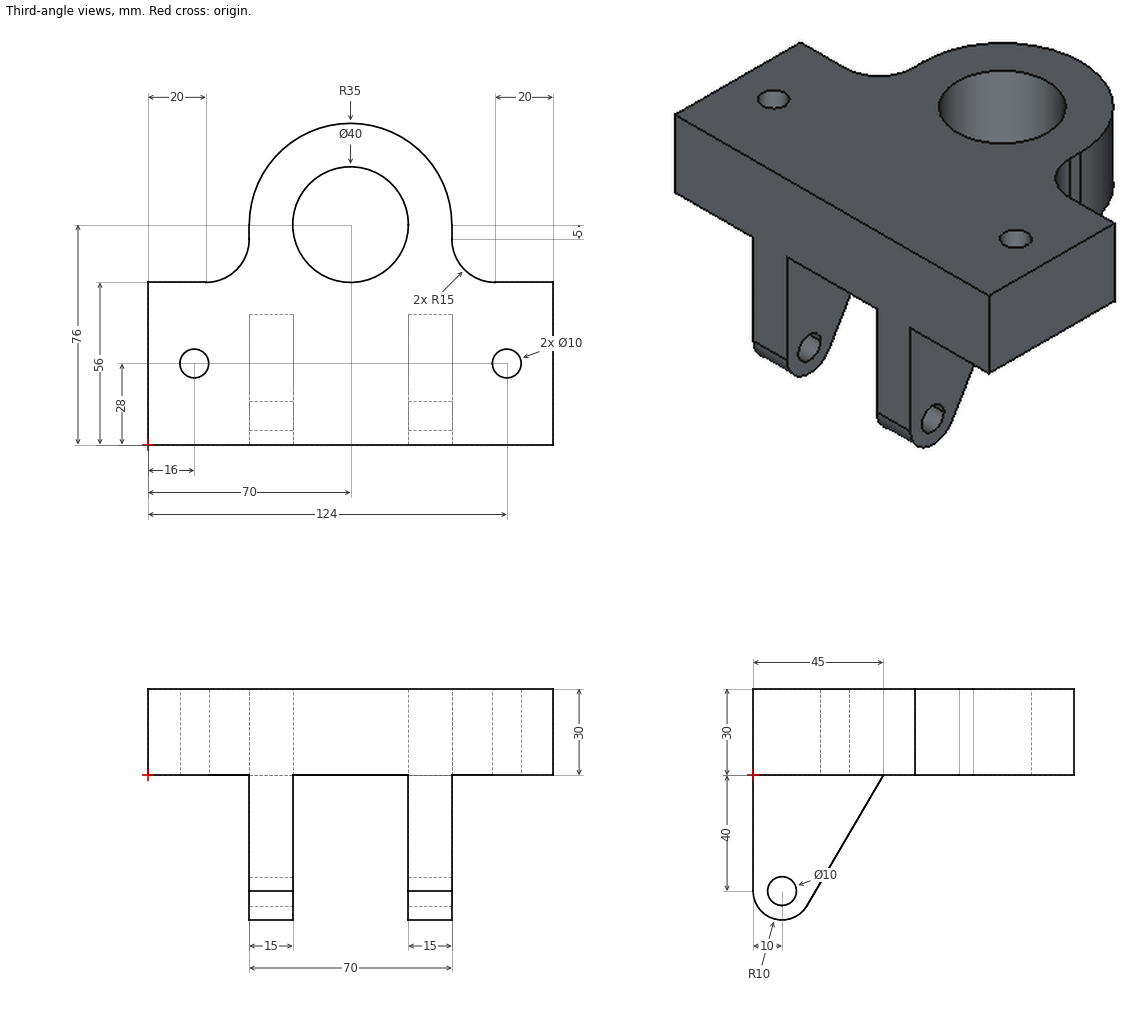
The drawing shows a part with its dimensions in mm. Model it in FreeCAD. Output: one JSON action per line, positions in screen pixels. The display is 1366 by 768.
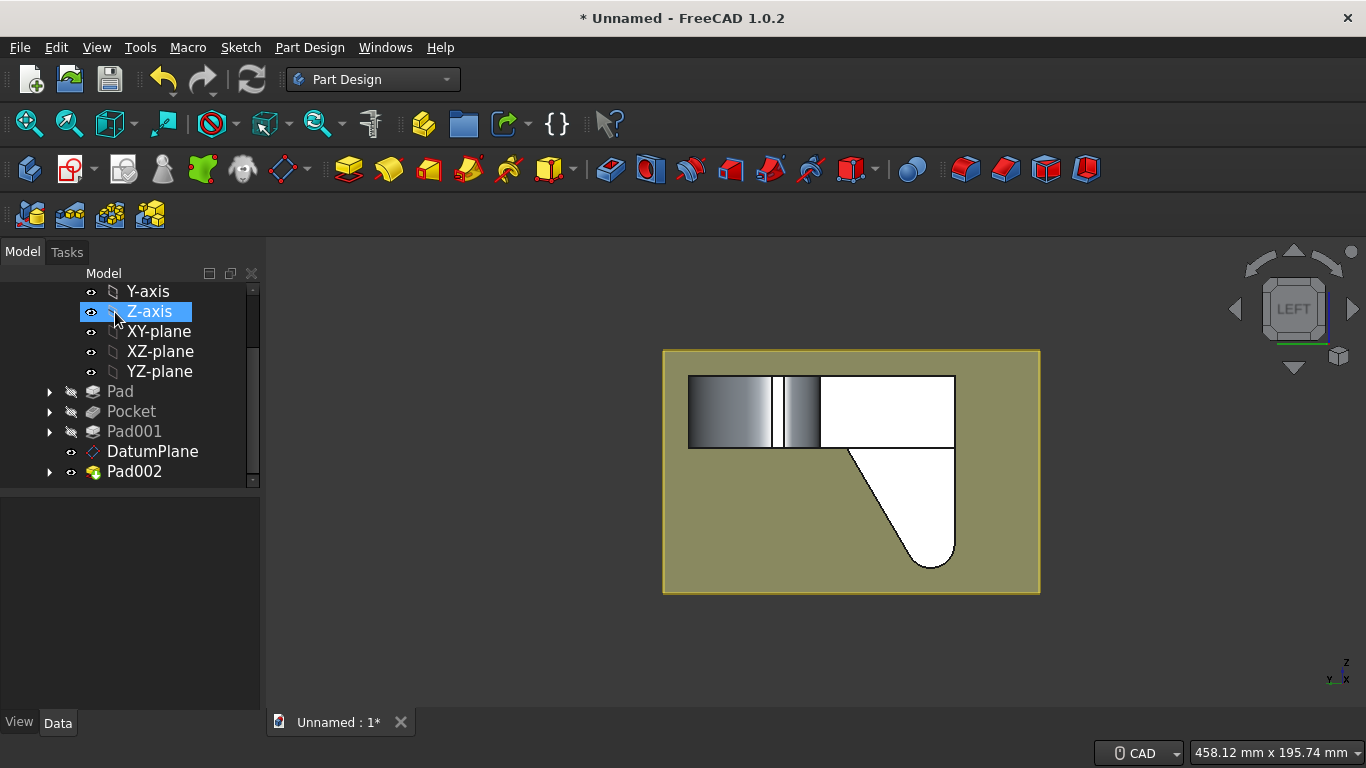
{"action": "left_click", "coordinate": [116, 452]}
{"action": "key", "text": "space"}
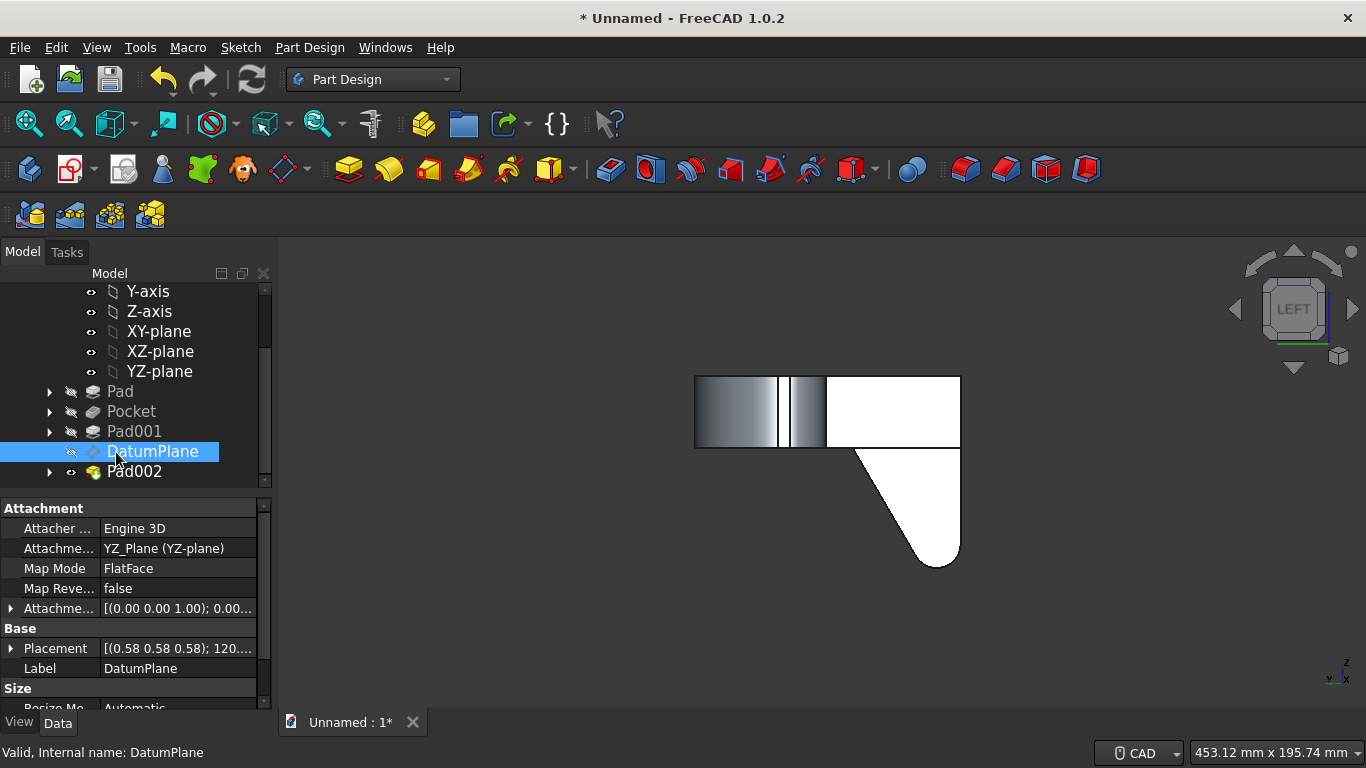
{"action": "left_click", "coordinate": [30, 124]}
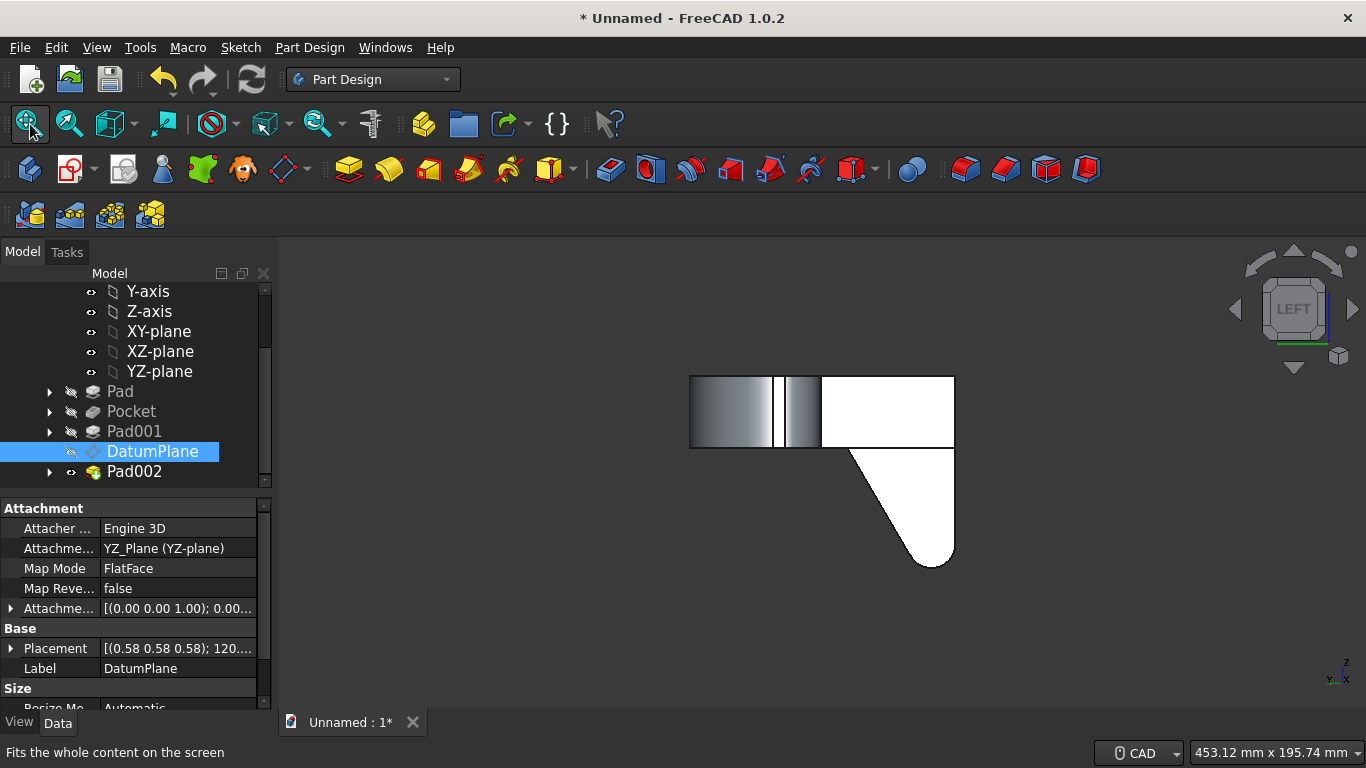
{"action": "key", "text": "0"}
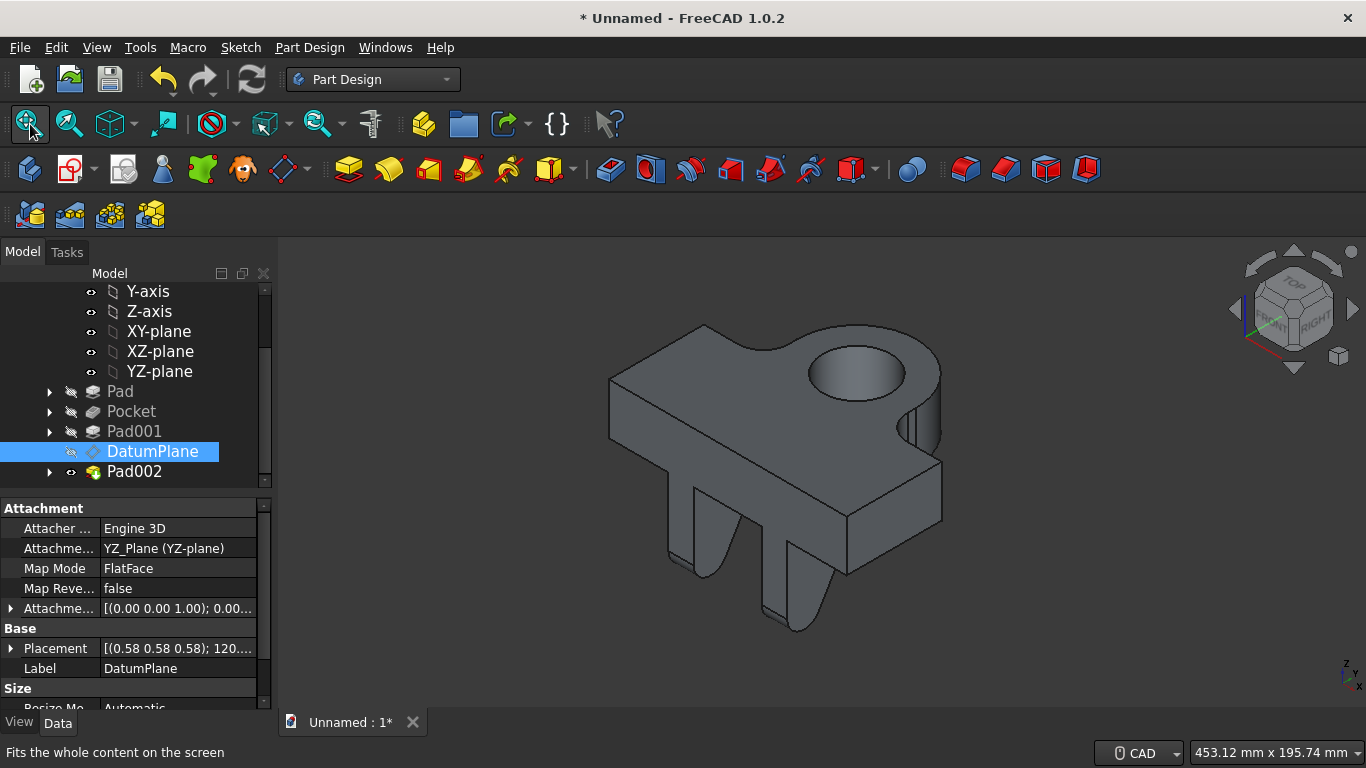
{"action": "left_click", "coordinate": [814, 573]}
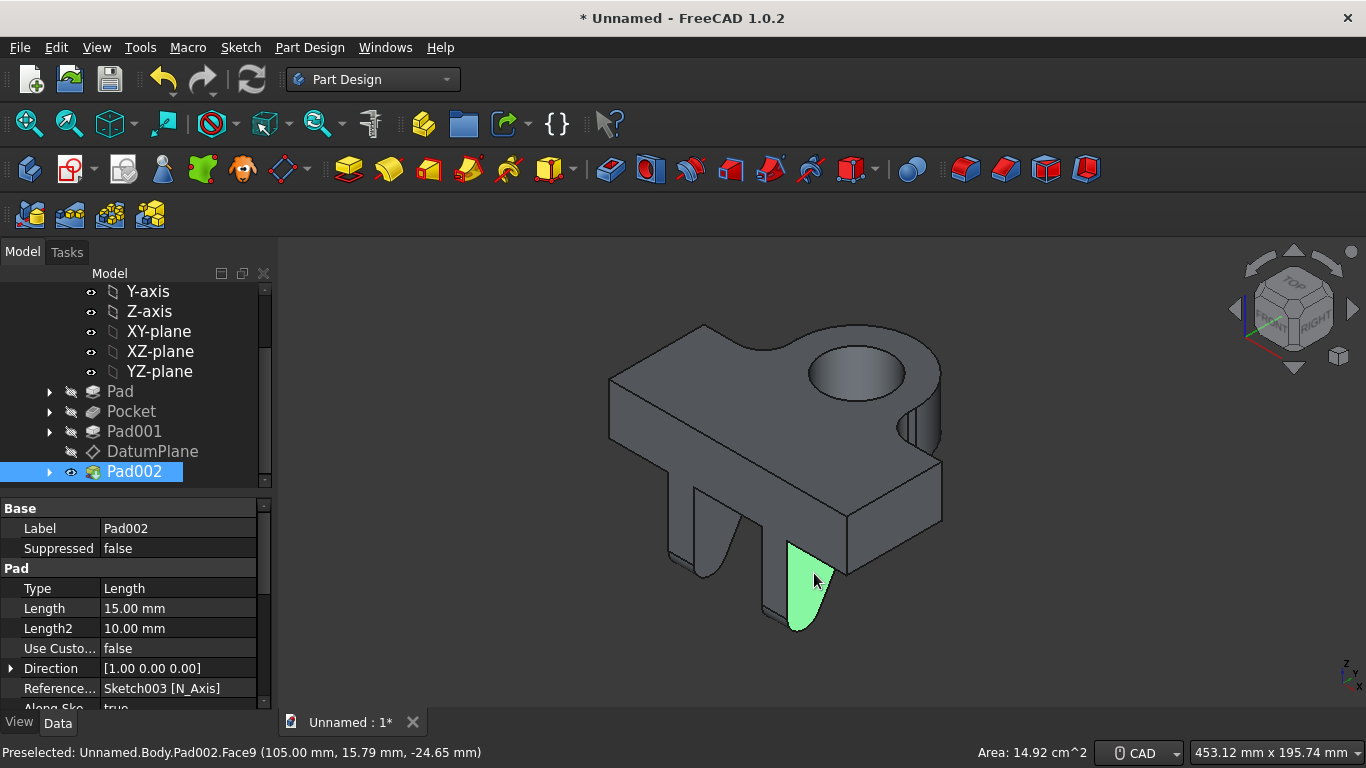
{"action": "left_click", "coordinate": [70, 170]}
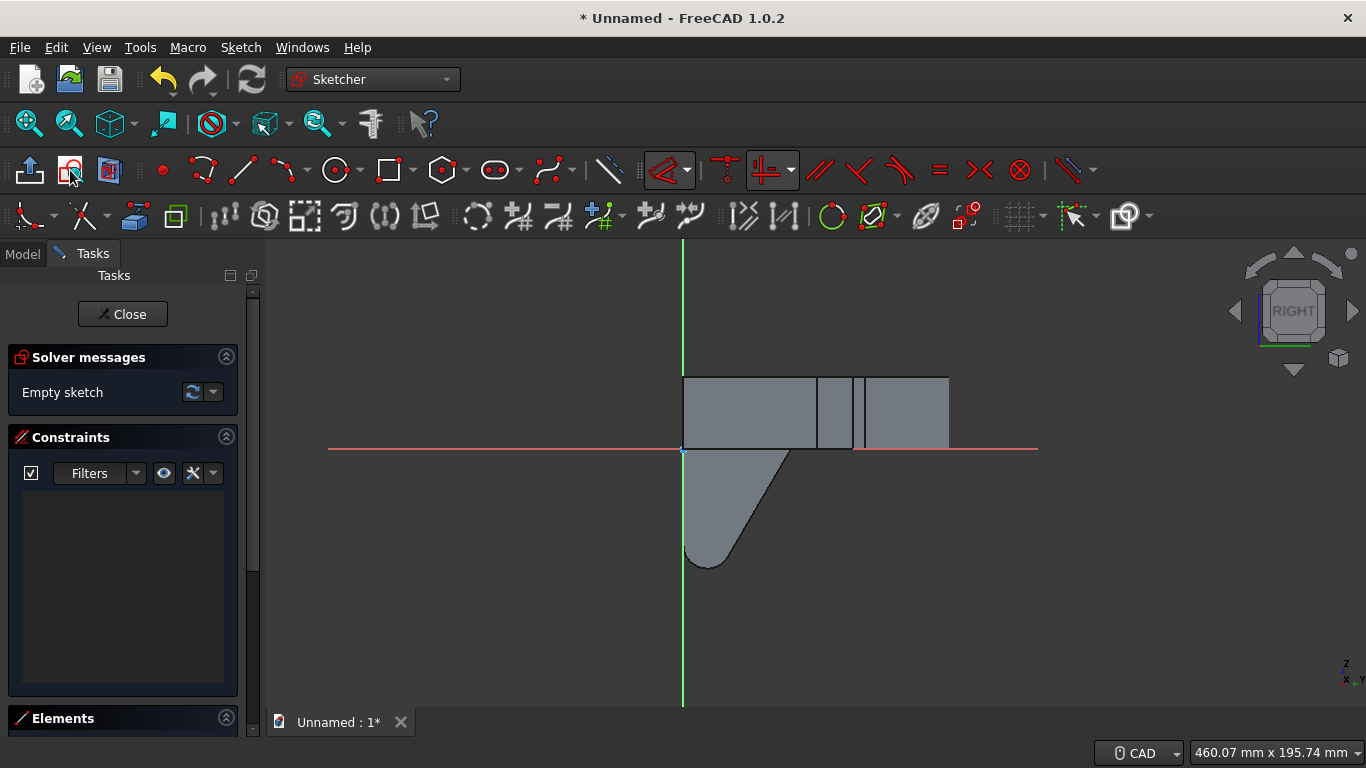
{"action": "scroll", "coordinate": [703, 552], "scroll_direction": "up", "scroll_amount": 12}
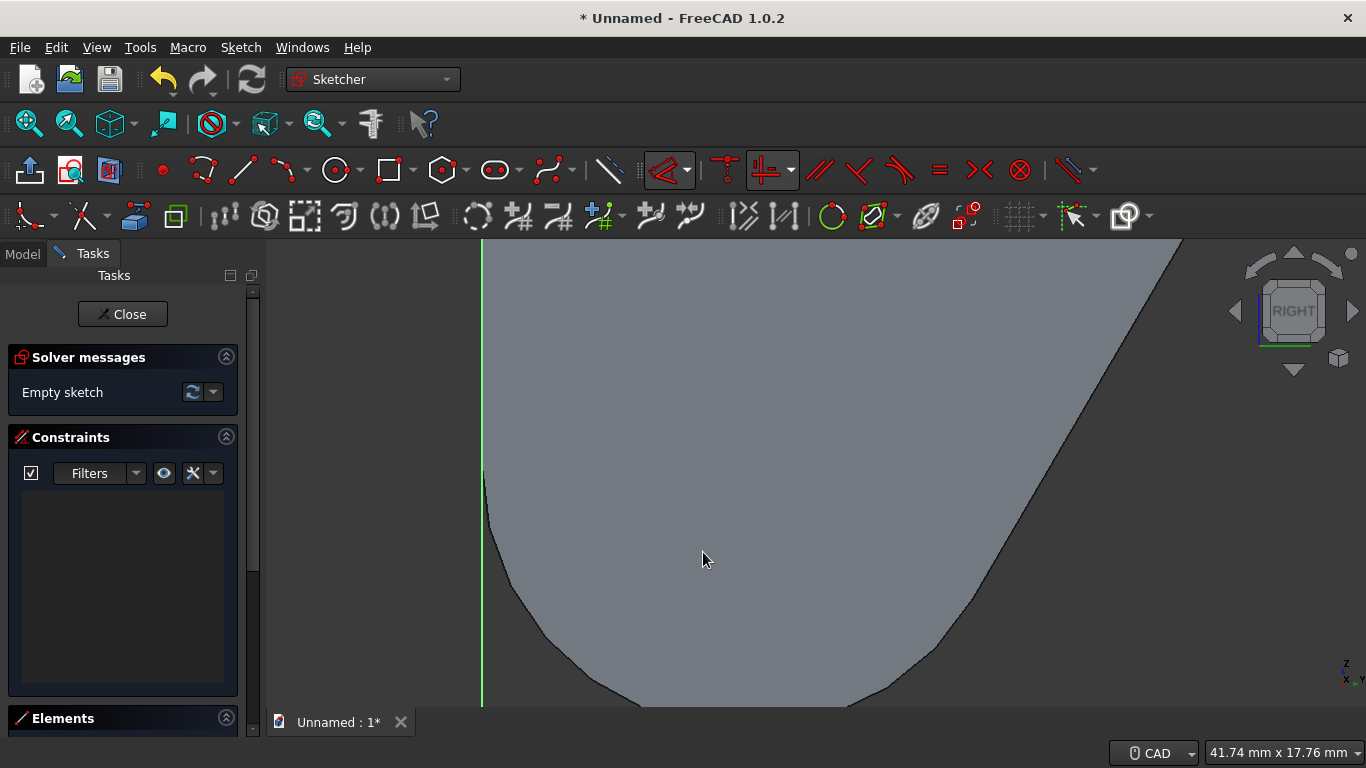
{"action": "key", "text": "g c"}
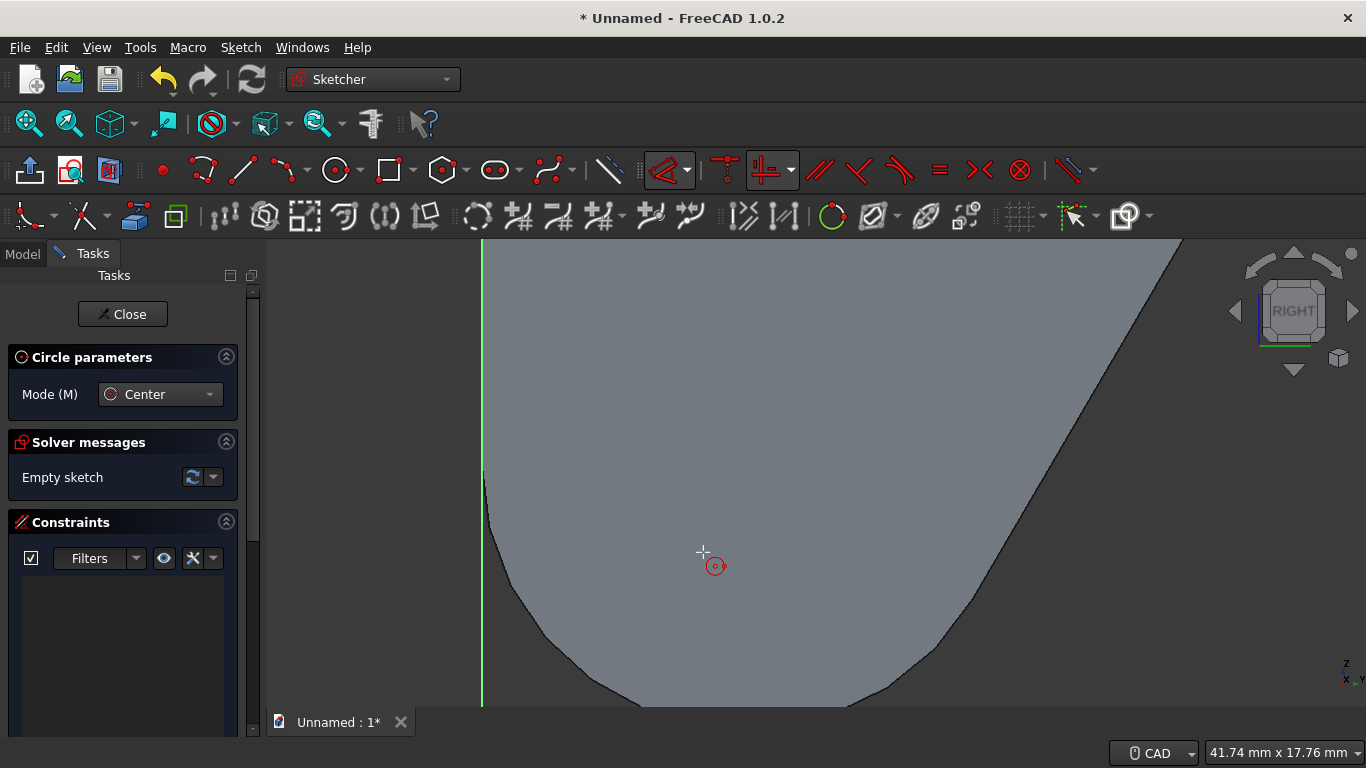
{"action": "left_click", "coordinate": [745, 466]}
{"action": "mouse_move", "coordinate": [839, 372]}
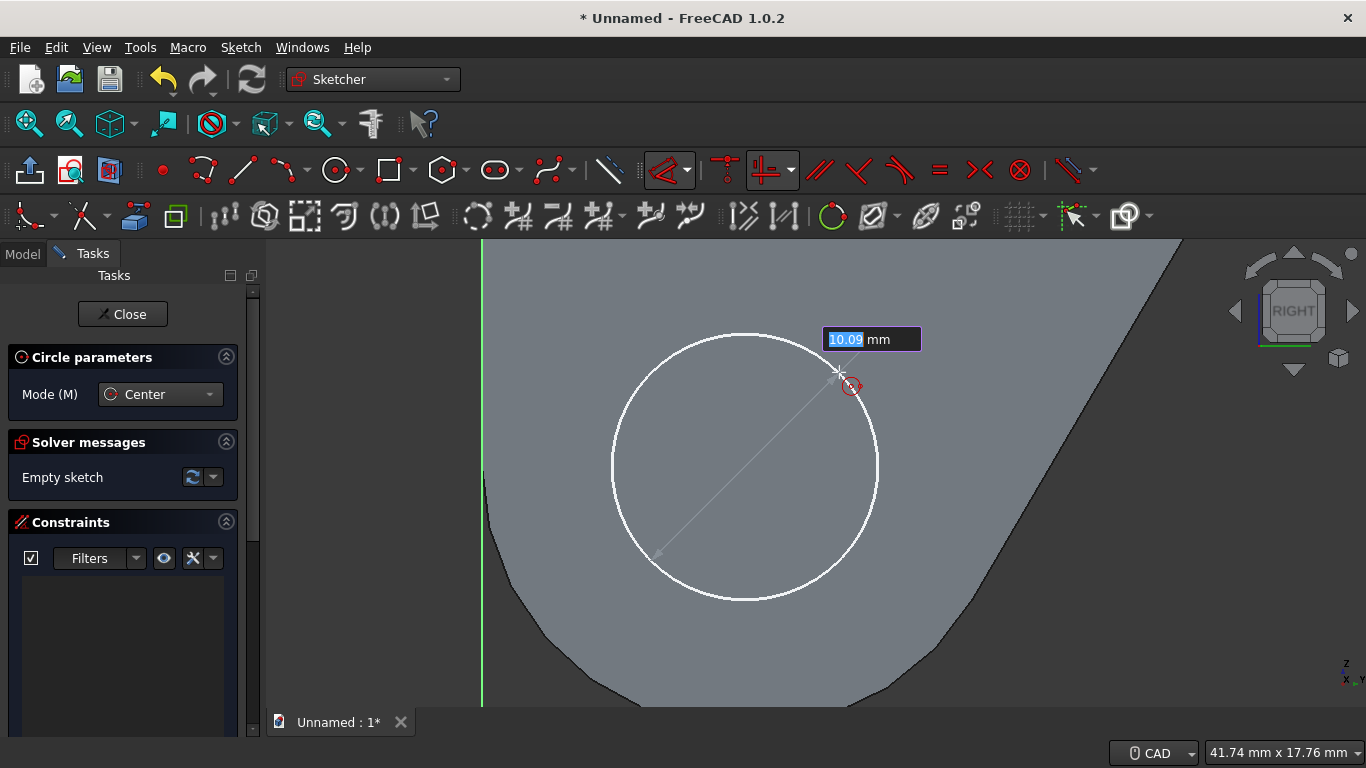
{"action": "type", "text": "10"}
{"action": "key", "text": "Return"}
{"action": "key", "text": "Escape"}